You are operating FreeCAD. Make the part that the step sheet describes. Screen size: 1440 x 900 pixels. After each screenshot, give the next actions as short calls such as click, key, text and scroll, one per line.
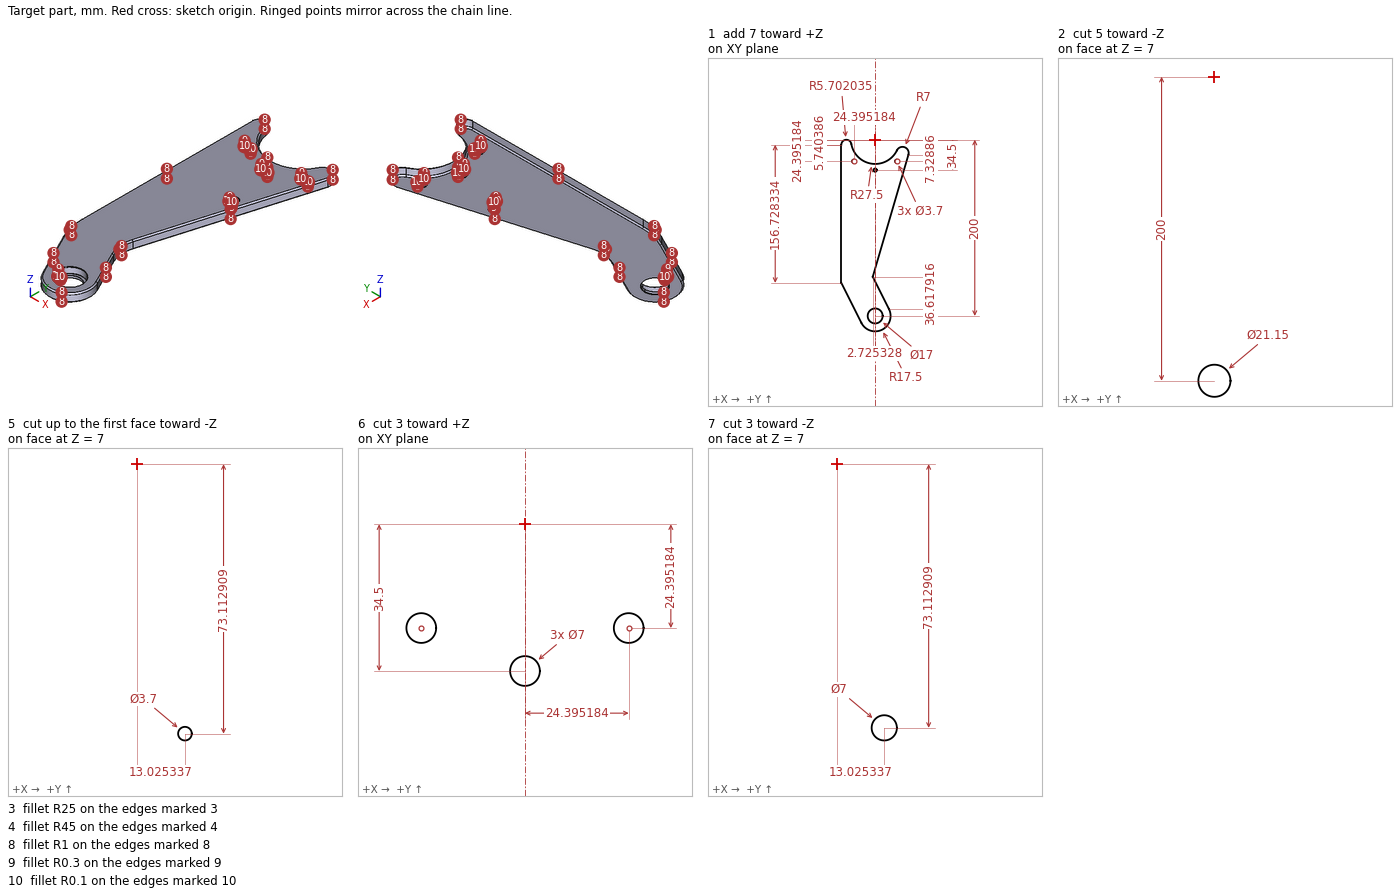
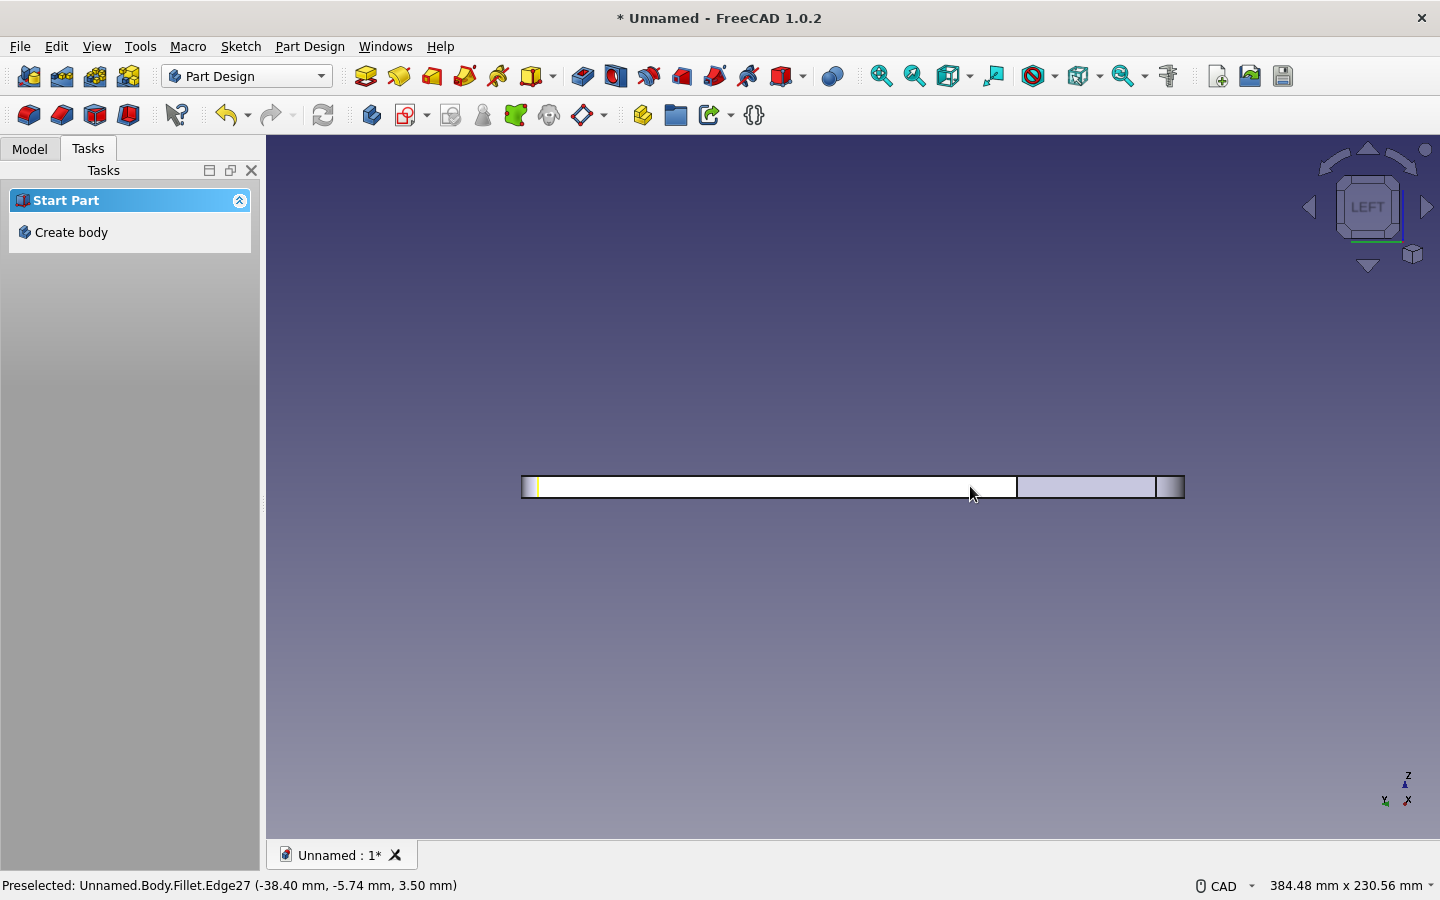
click(1017, 486)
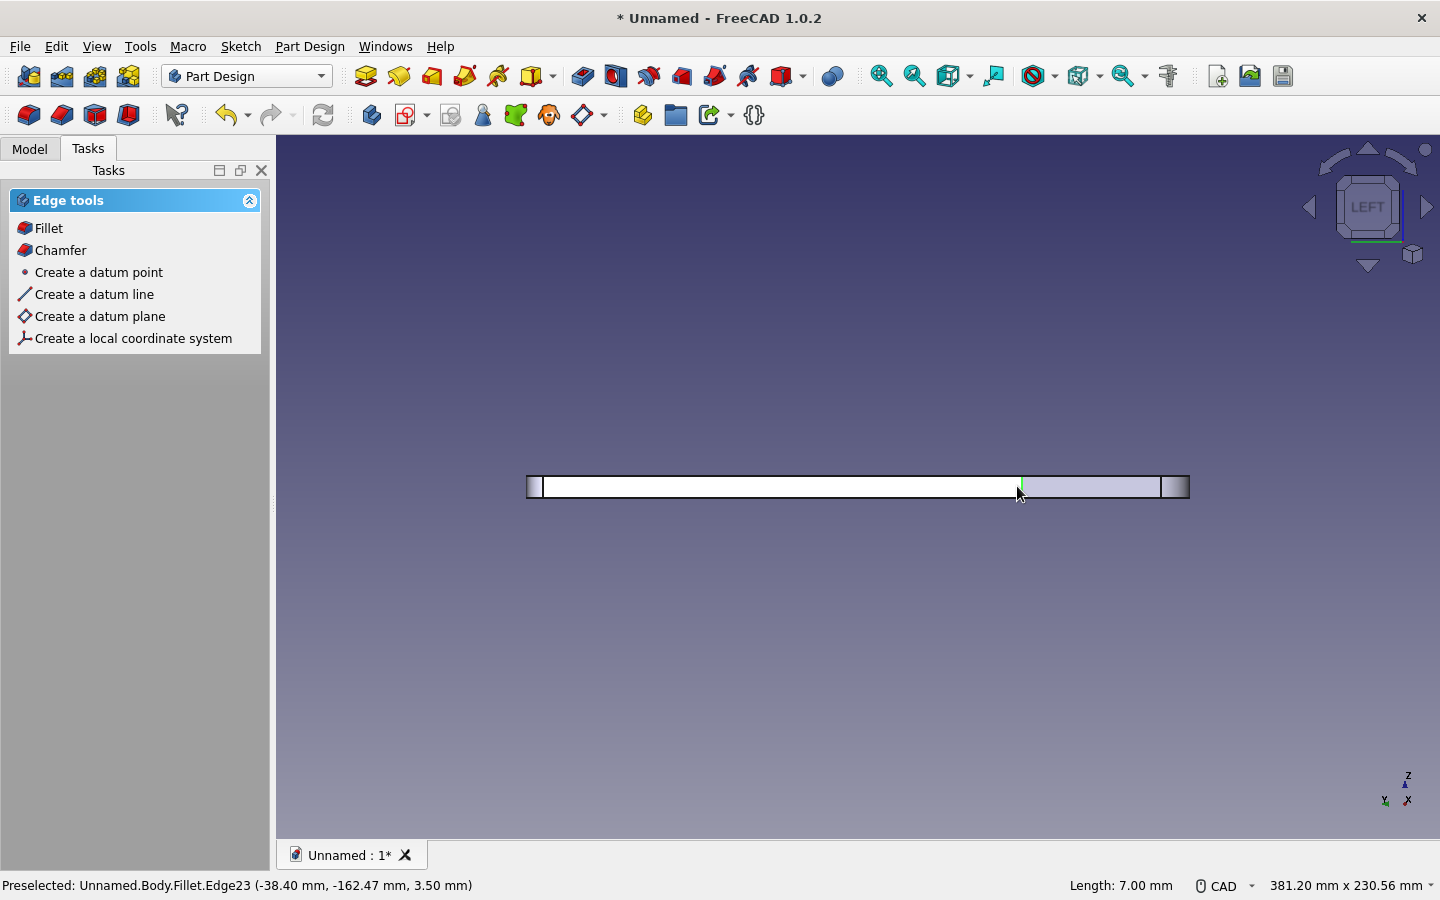
click(29, 116)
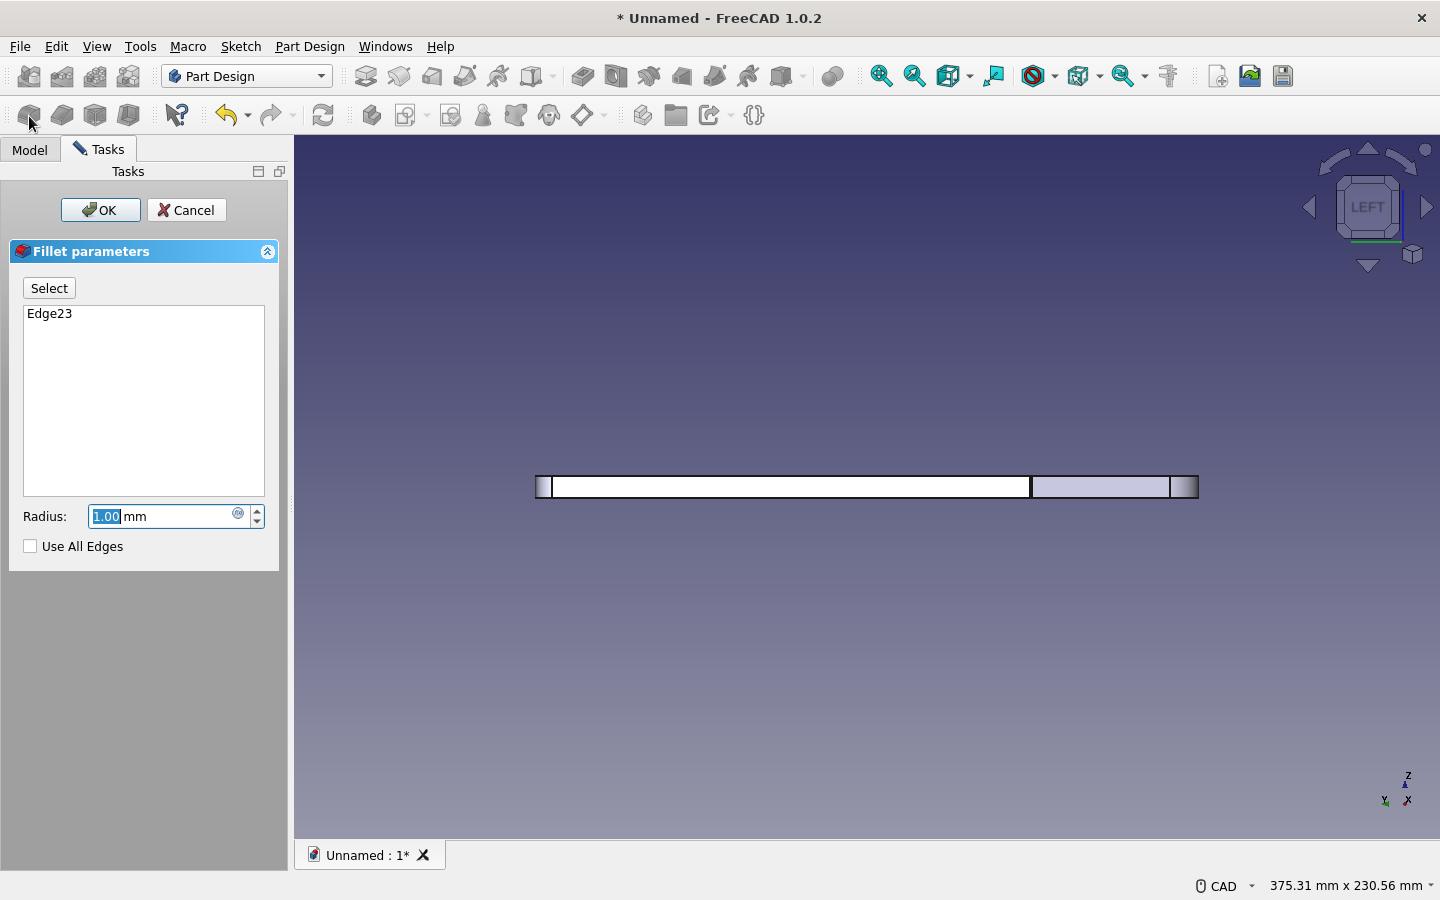
text(45)
key(Tab)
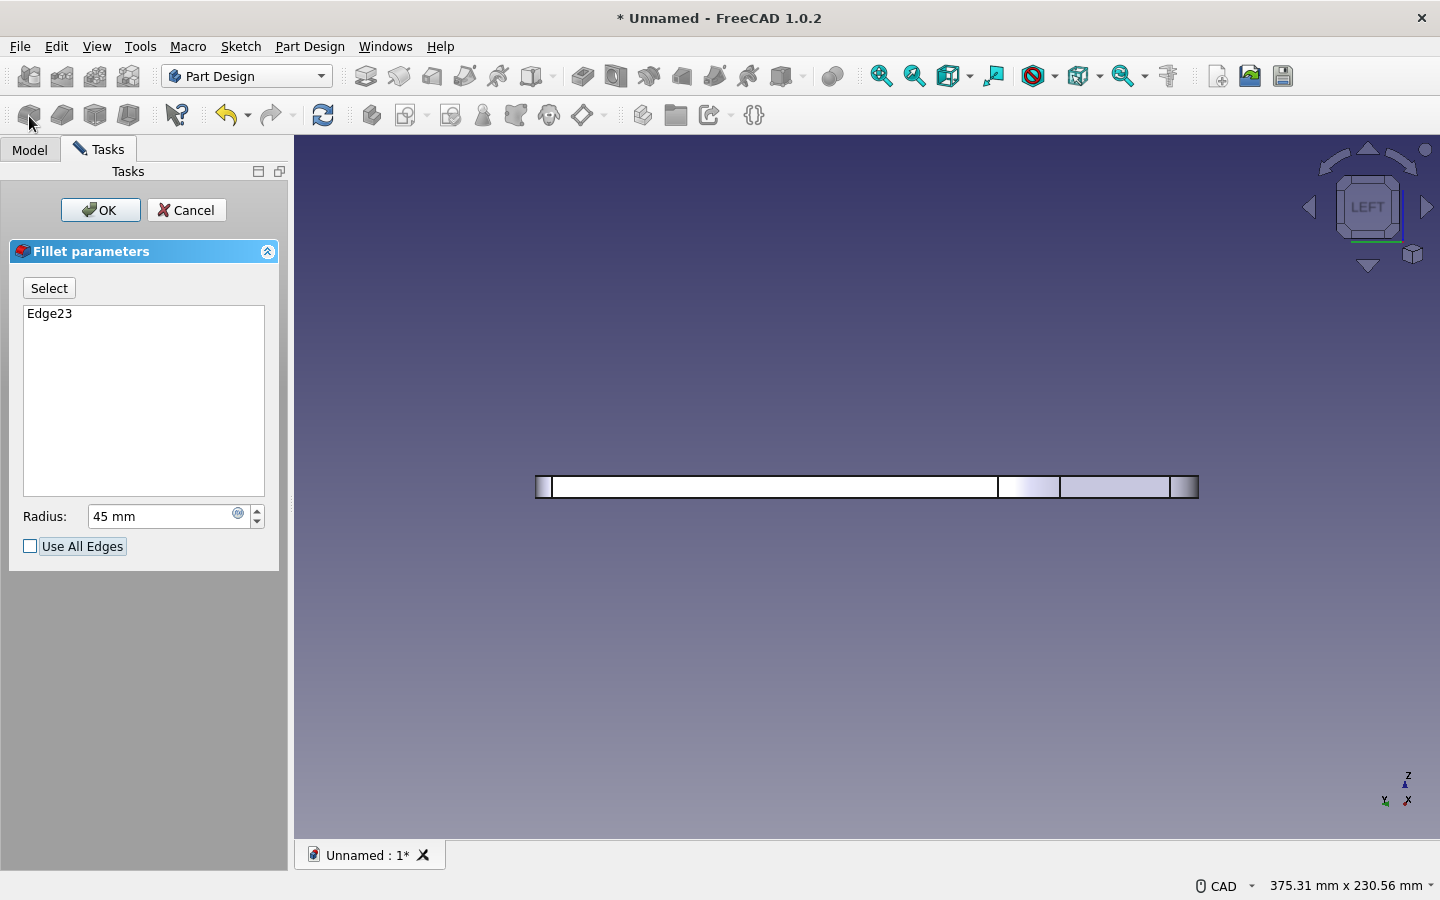
click(101, 210)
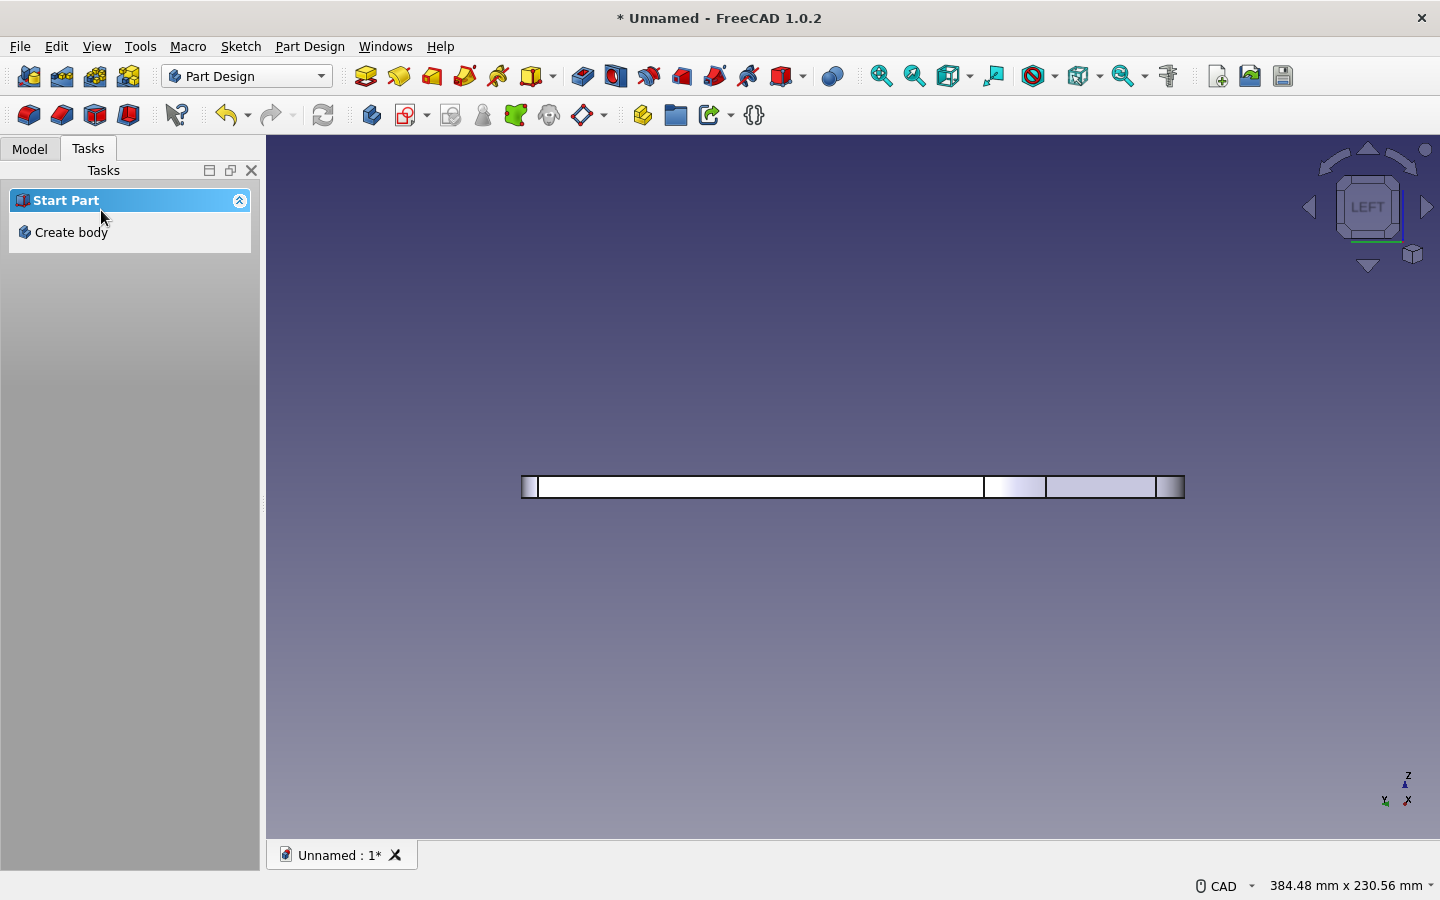
key(0)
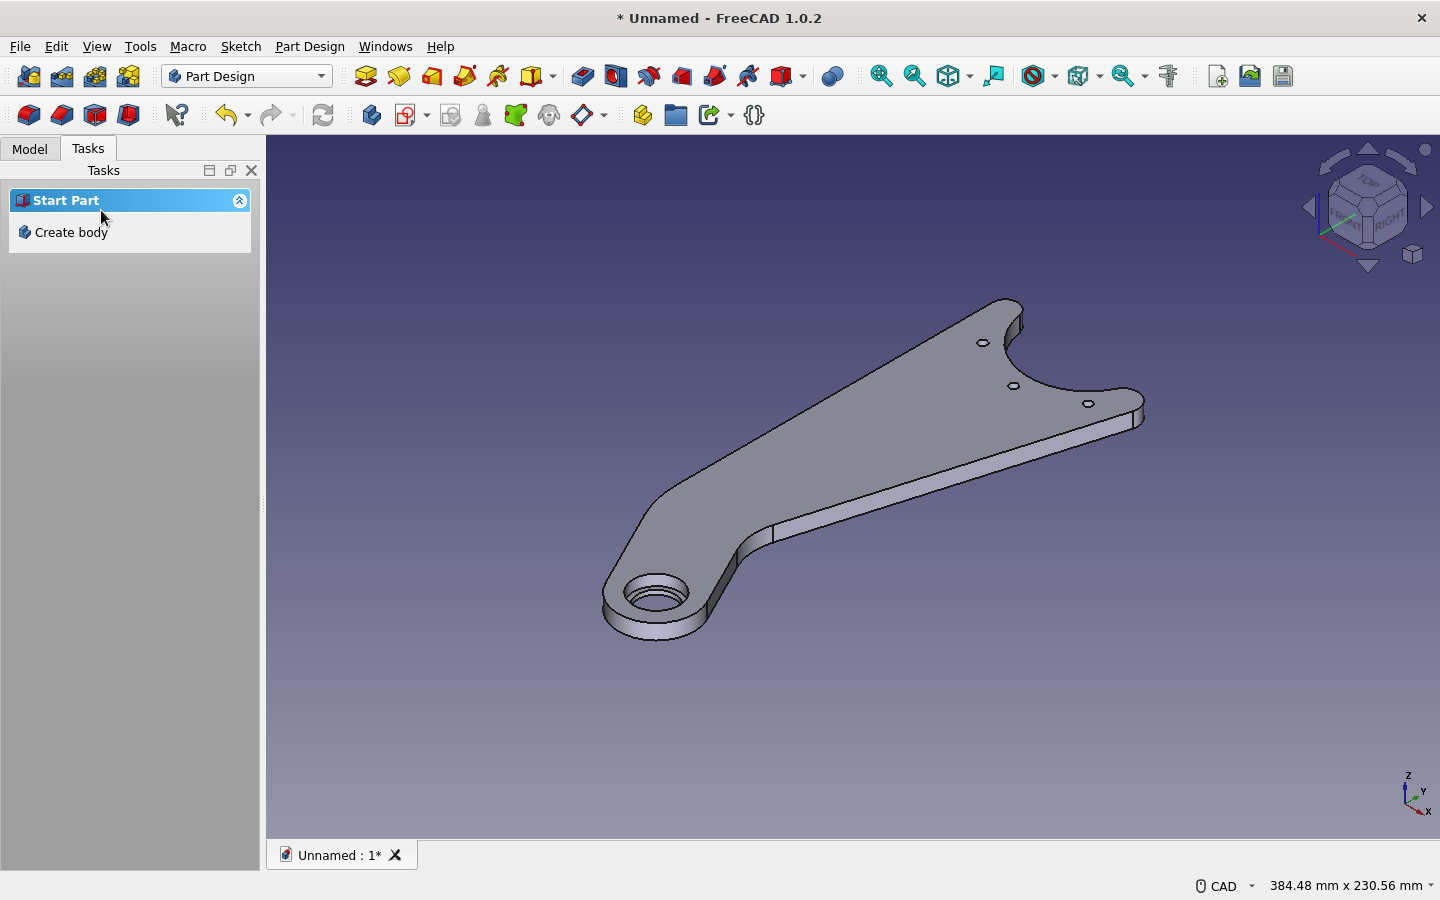
click(896, 425)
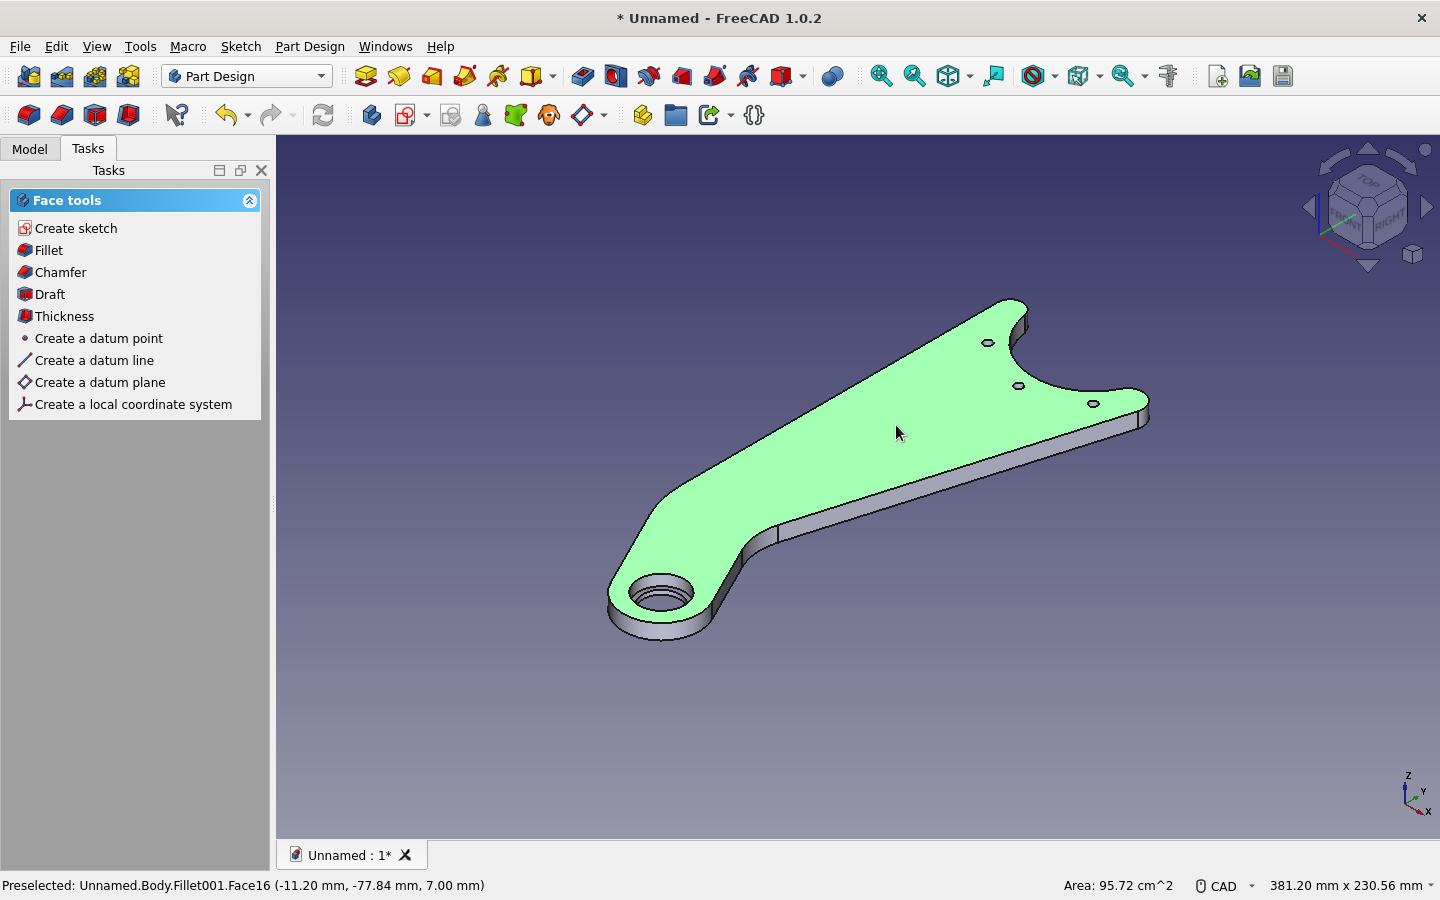
click(404, 116)